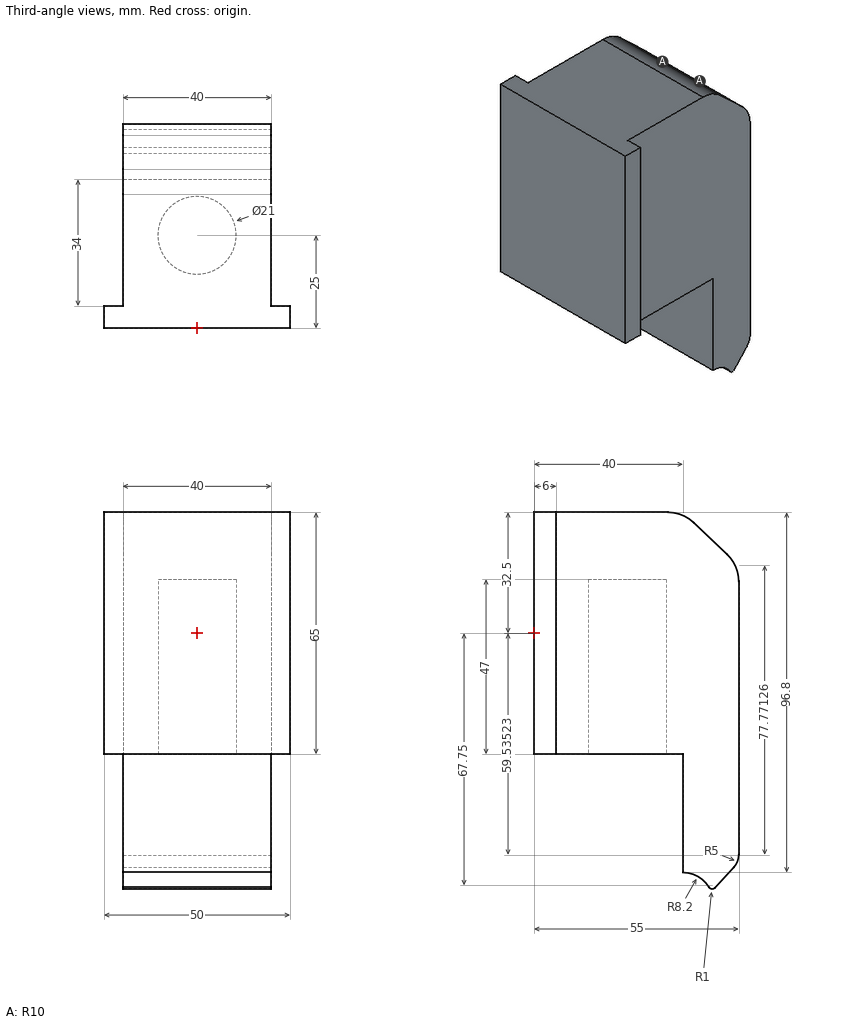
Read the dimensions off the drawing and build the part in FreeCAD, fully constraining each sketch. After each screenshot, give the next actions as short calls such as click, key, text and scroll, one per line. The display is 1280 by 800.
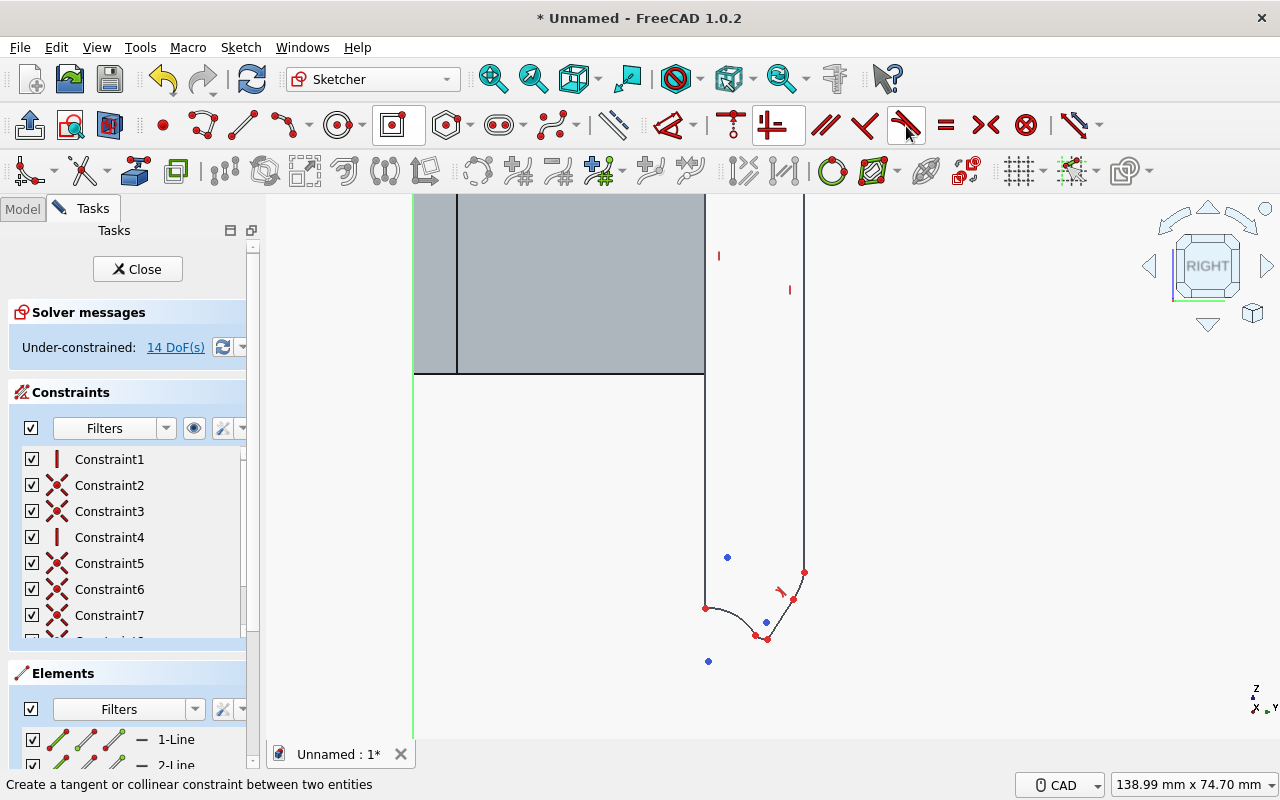
click(776, 627)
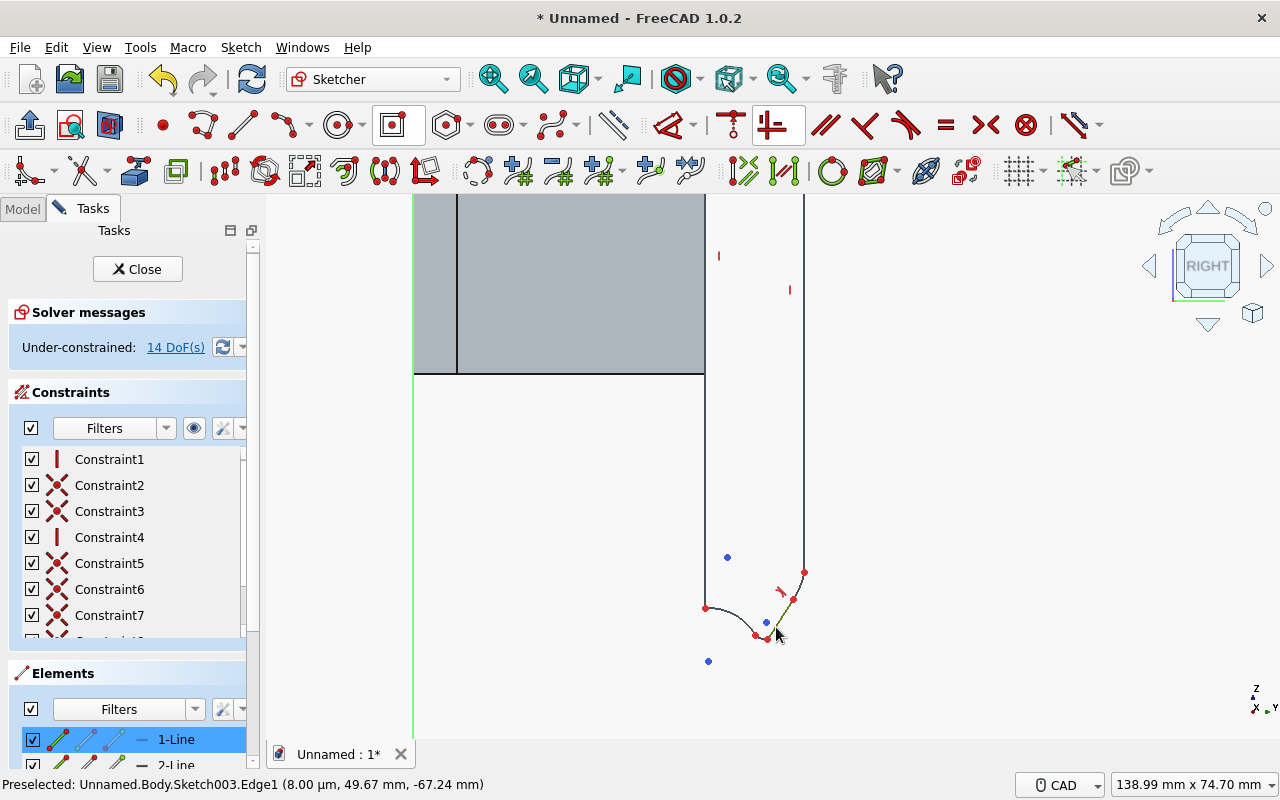
scroll(762, 639, up, 4)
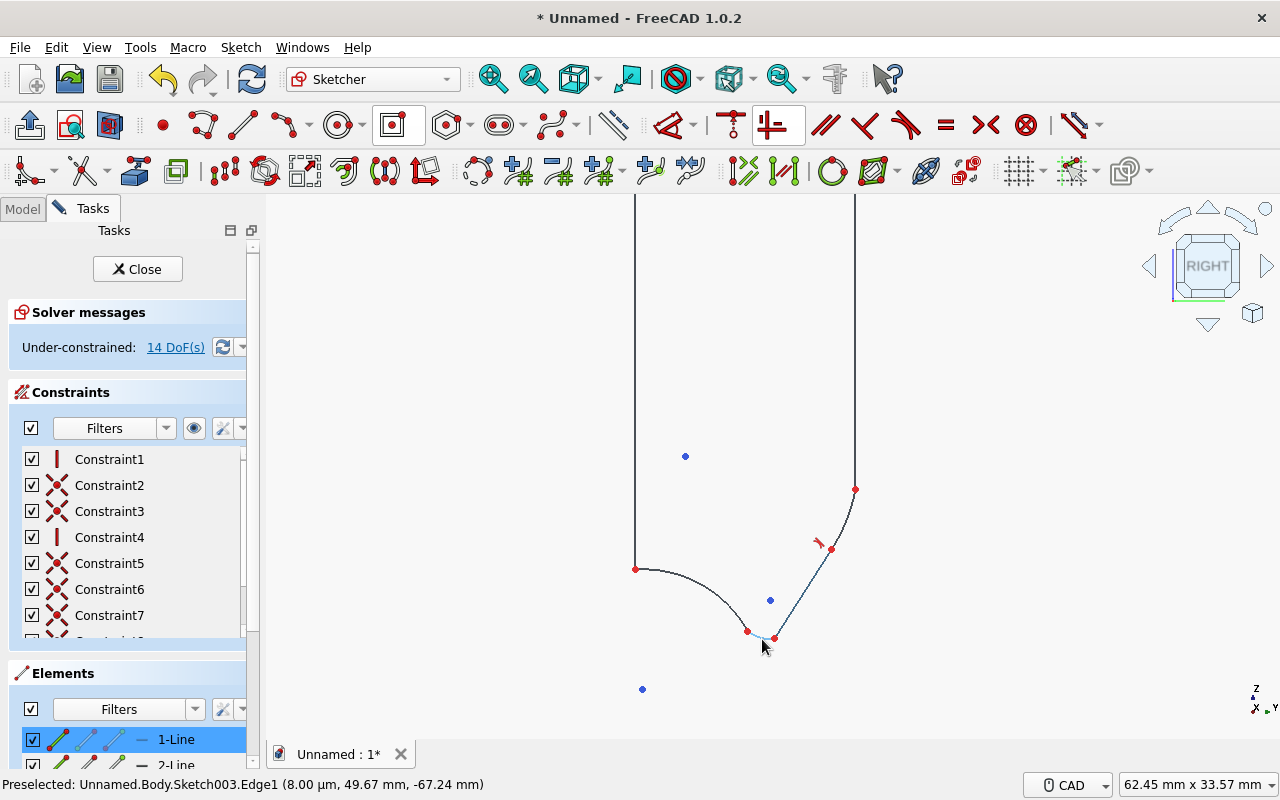
click(760, 638)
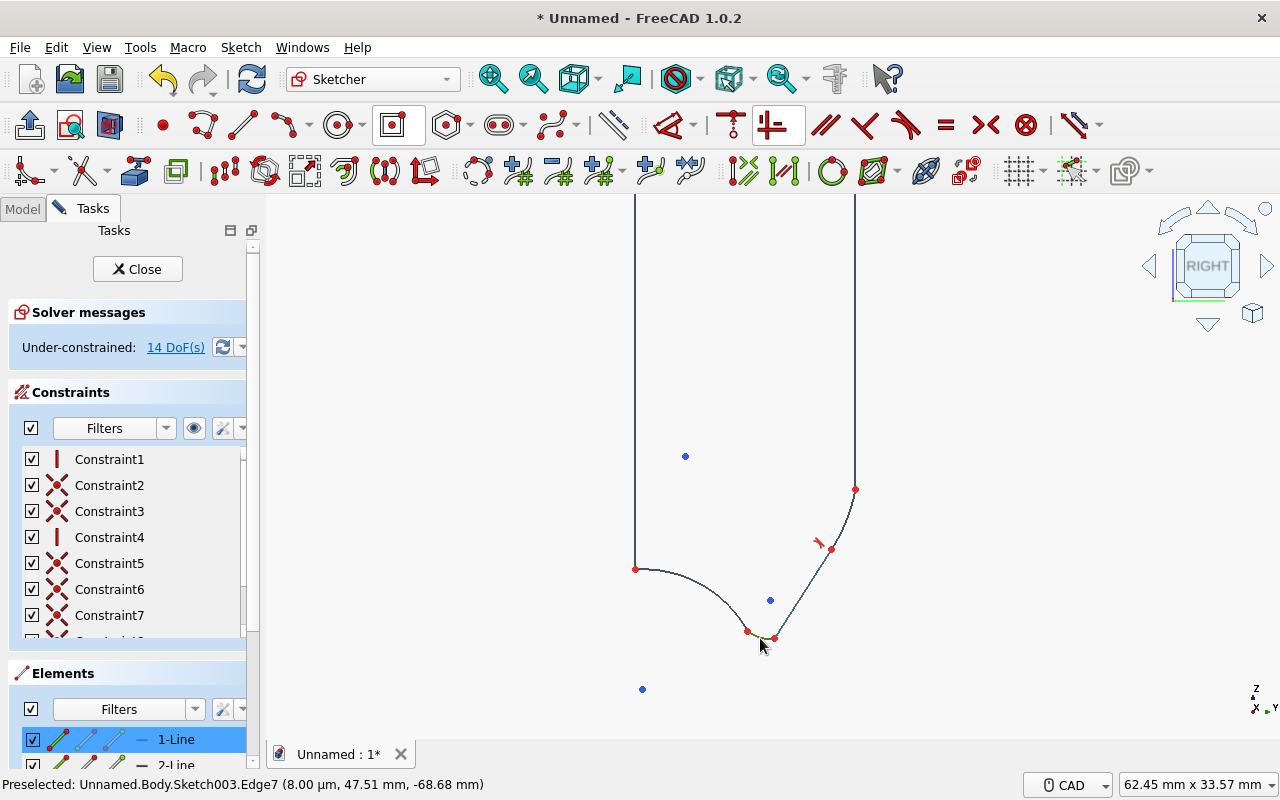
click(906, 126)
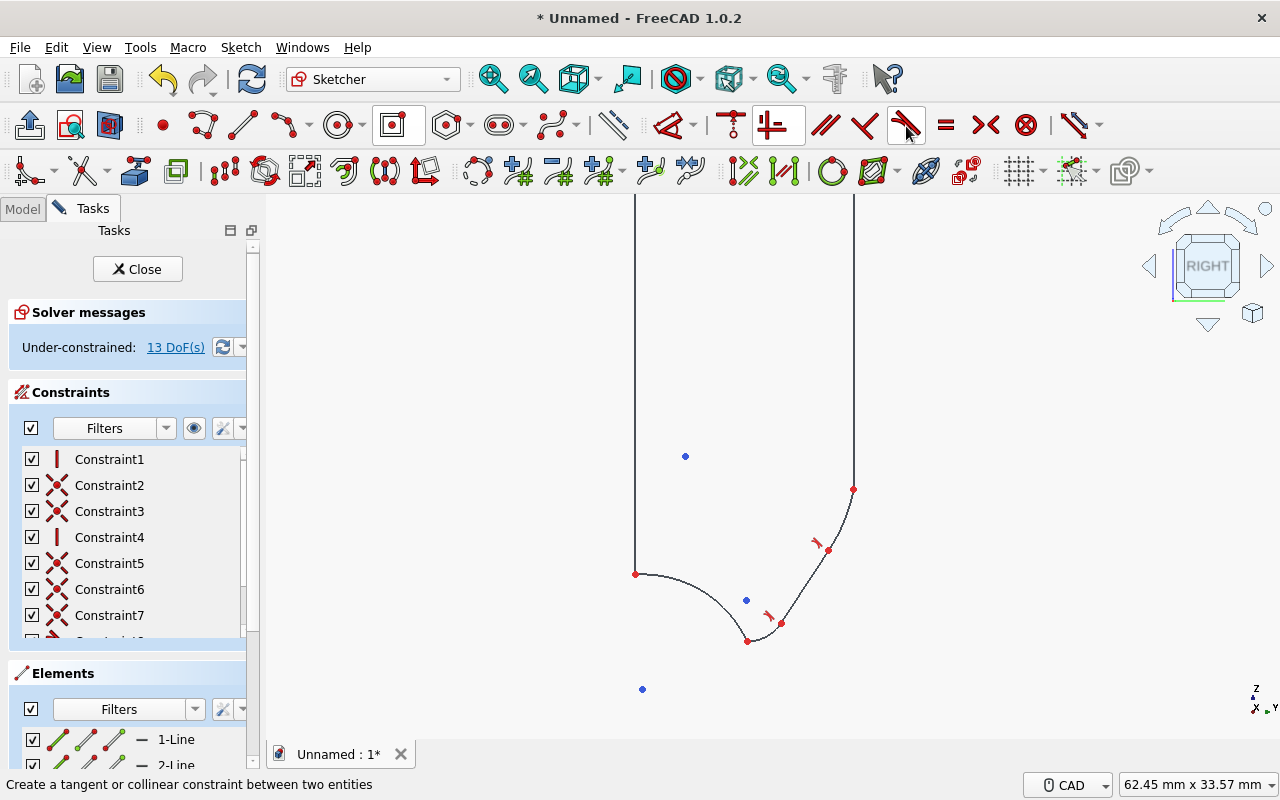
scroll(774, 631, down, 8)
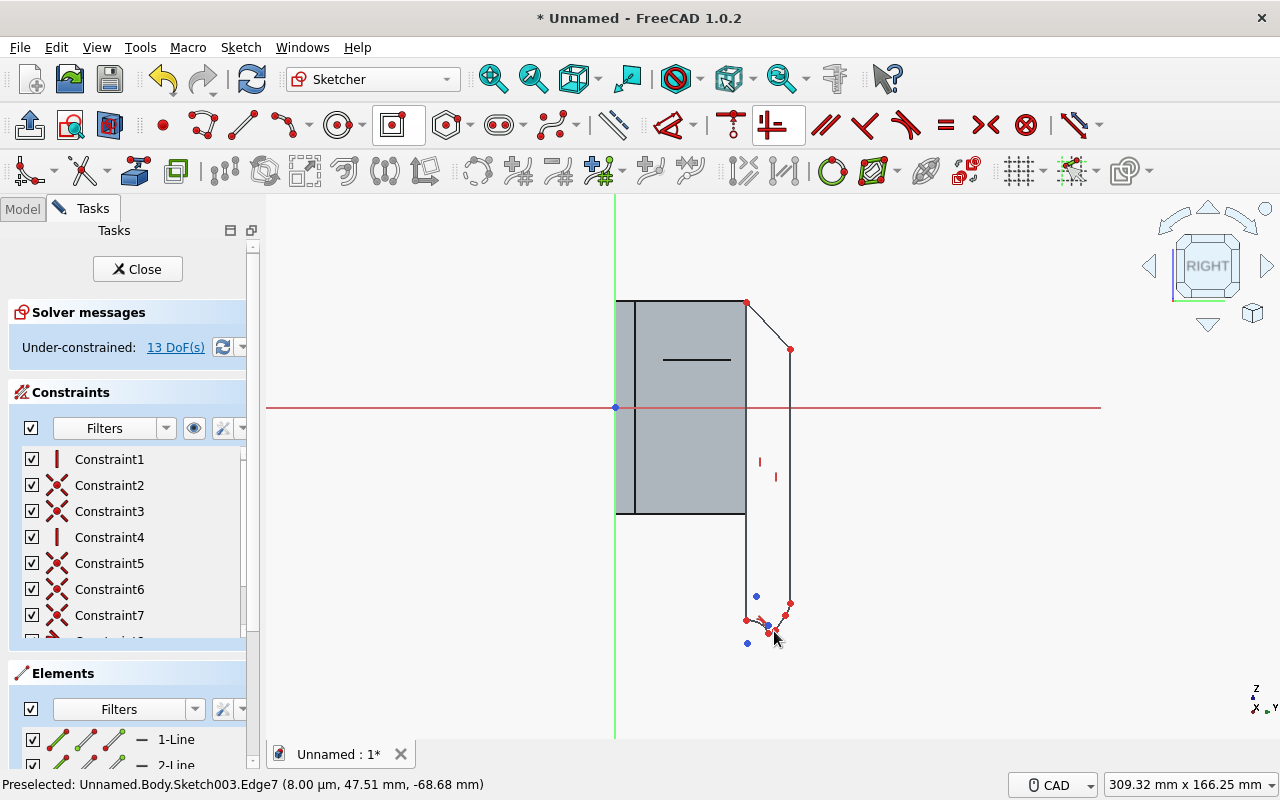
click(790, 552)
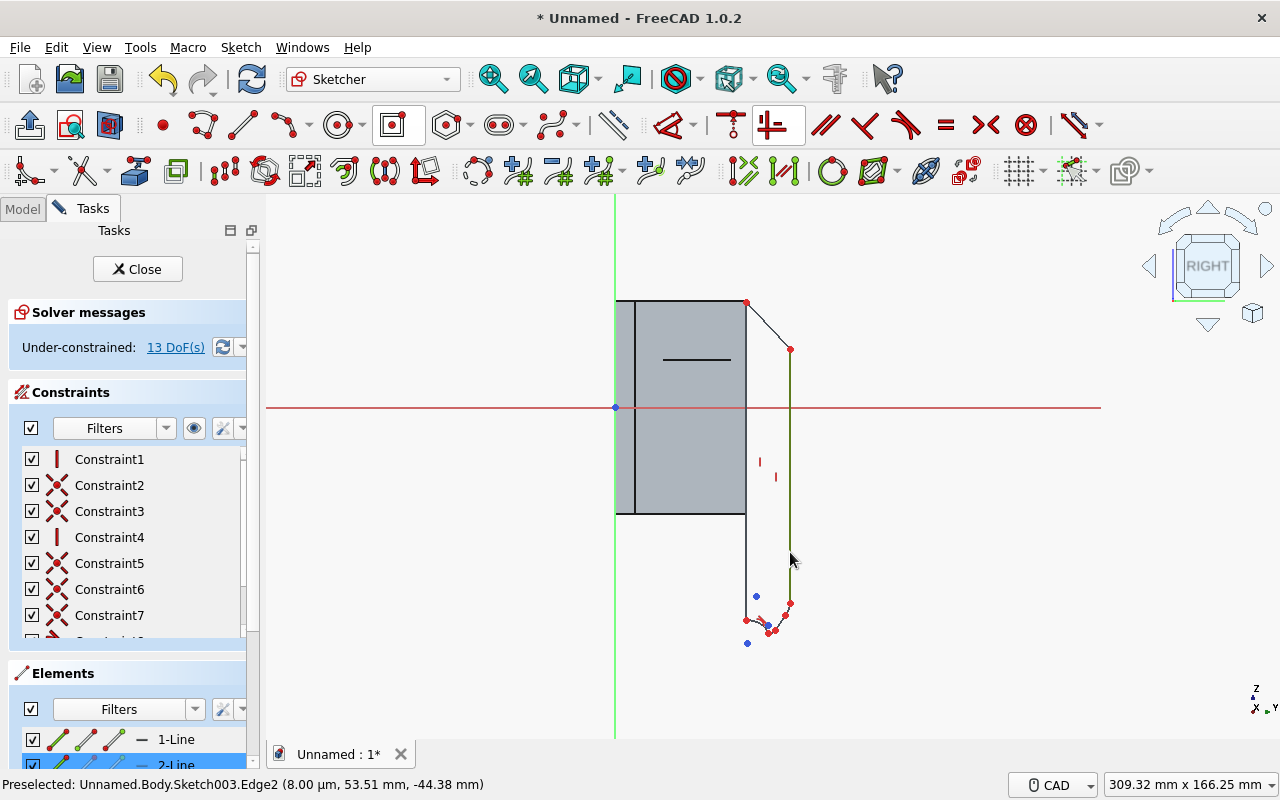
scroll(789, 610, up, 4)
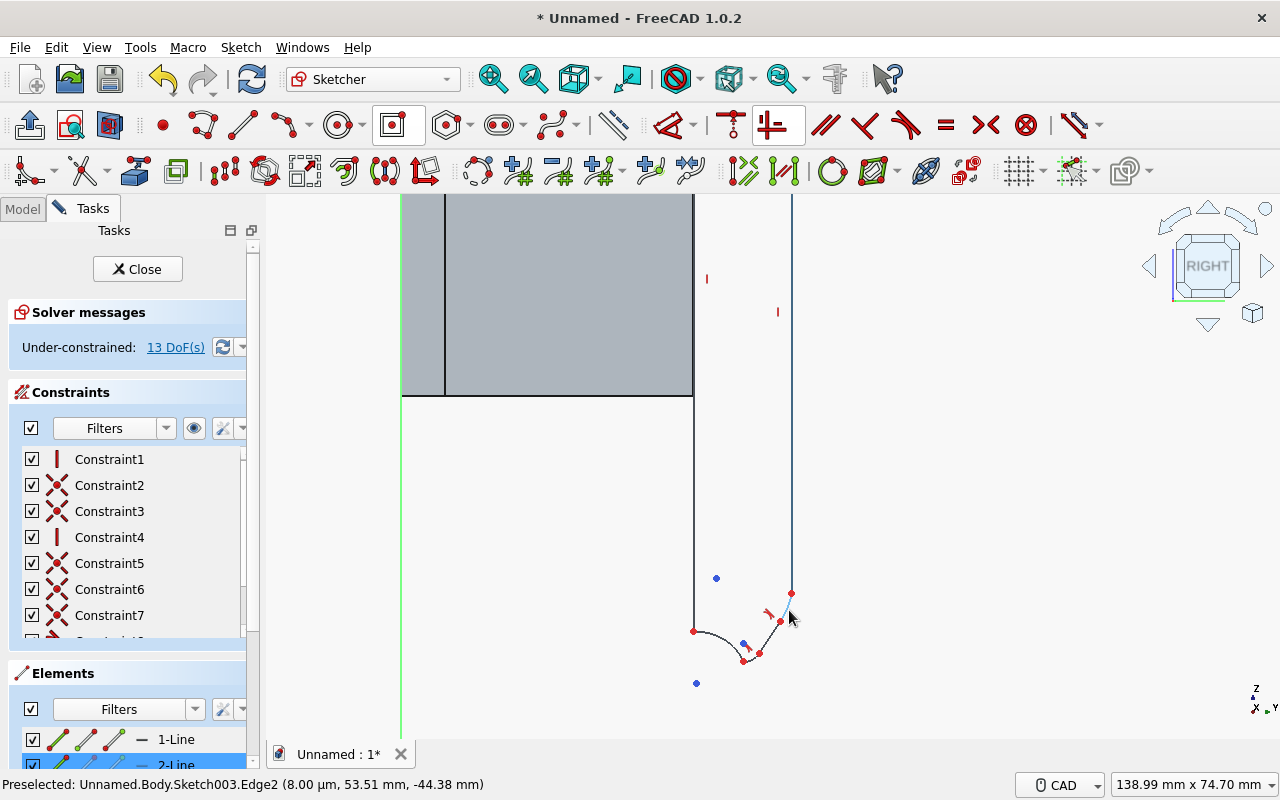
click(787, 608)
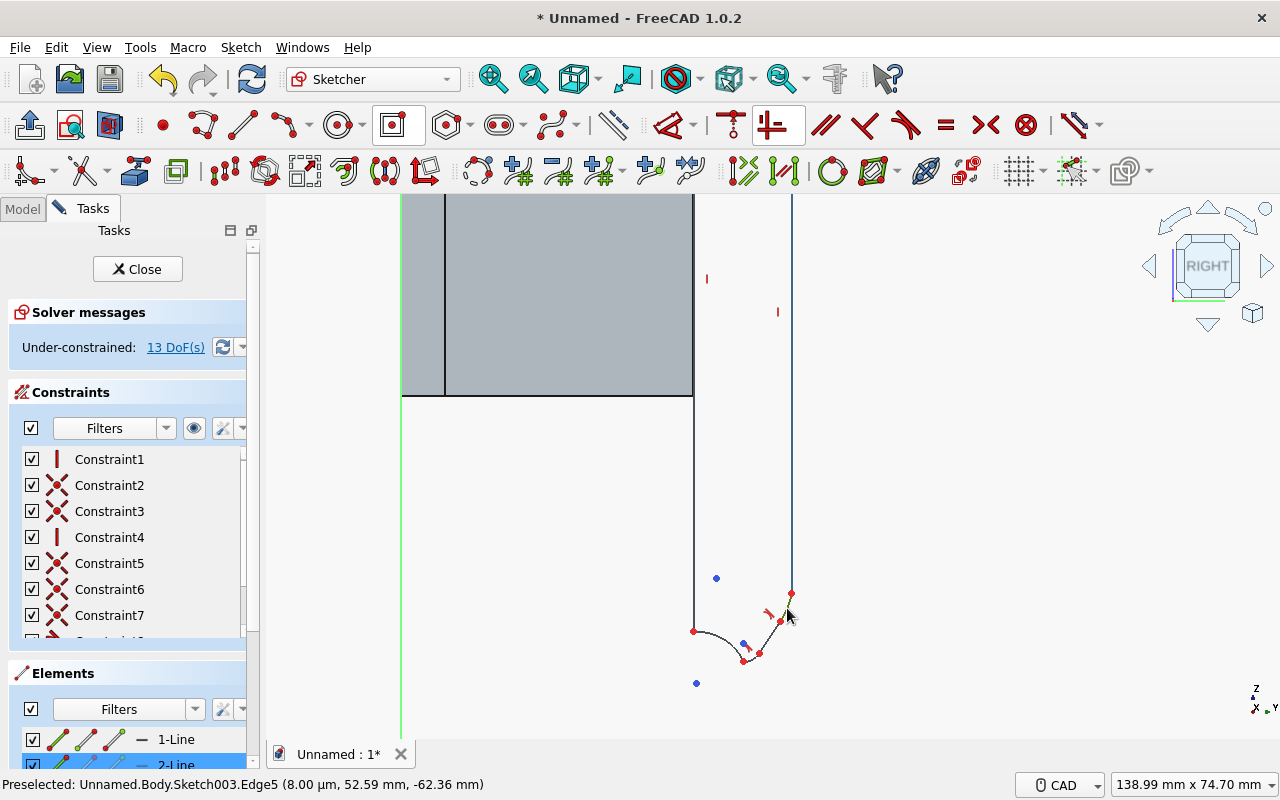
click(906, 126)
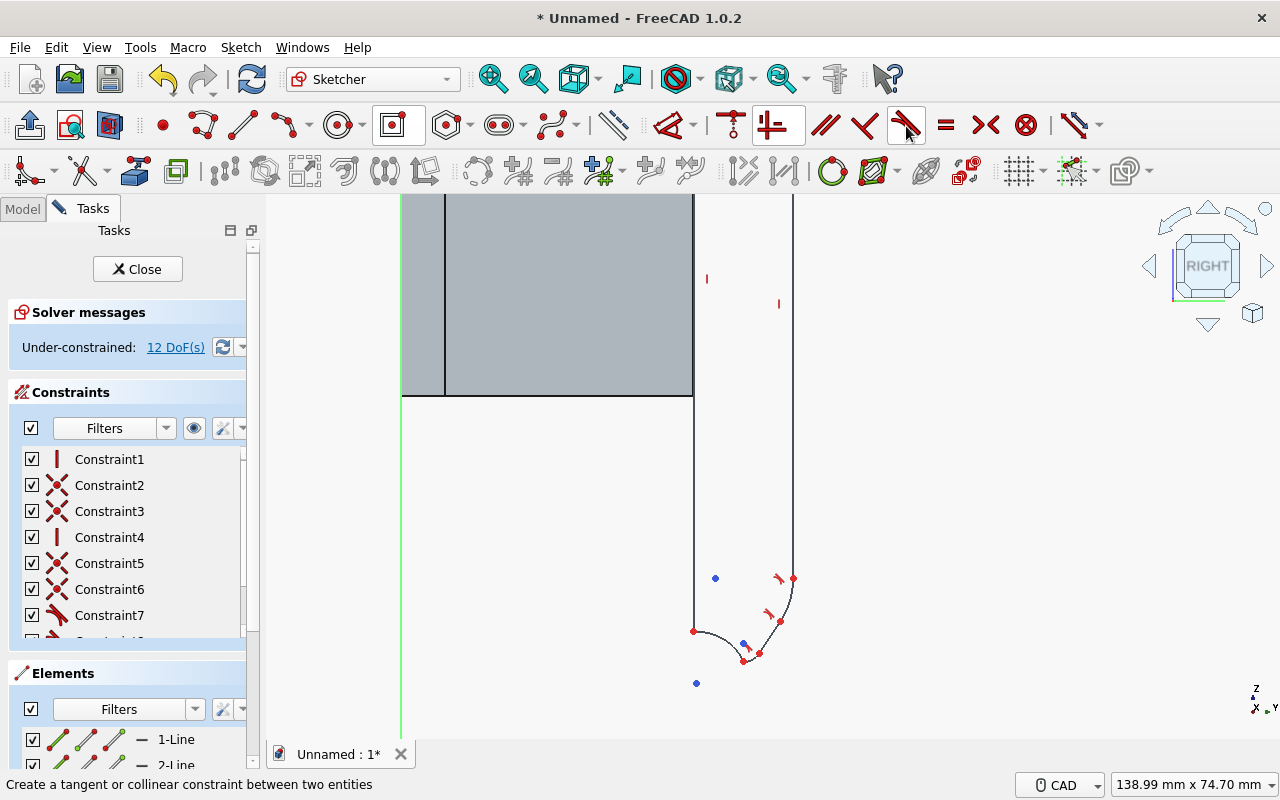
click(733, 647)